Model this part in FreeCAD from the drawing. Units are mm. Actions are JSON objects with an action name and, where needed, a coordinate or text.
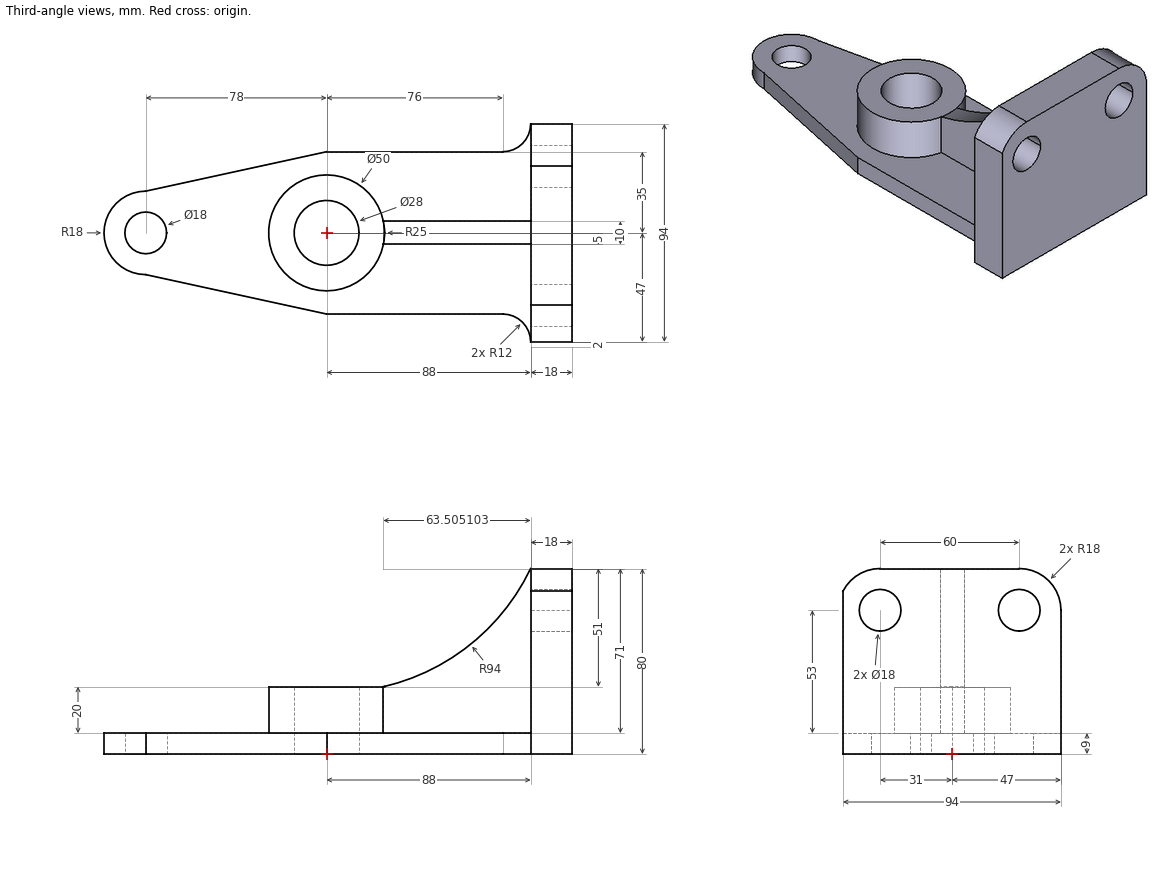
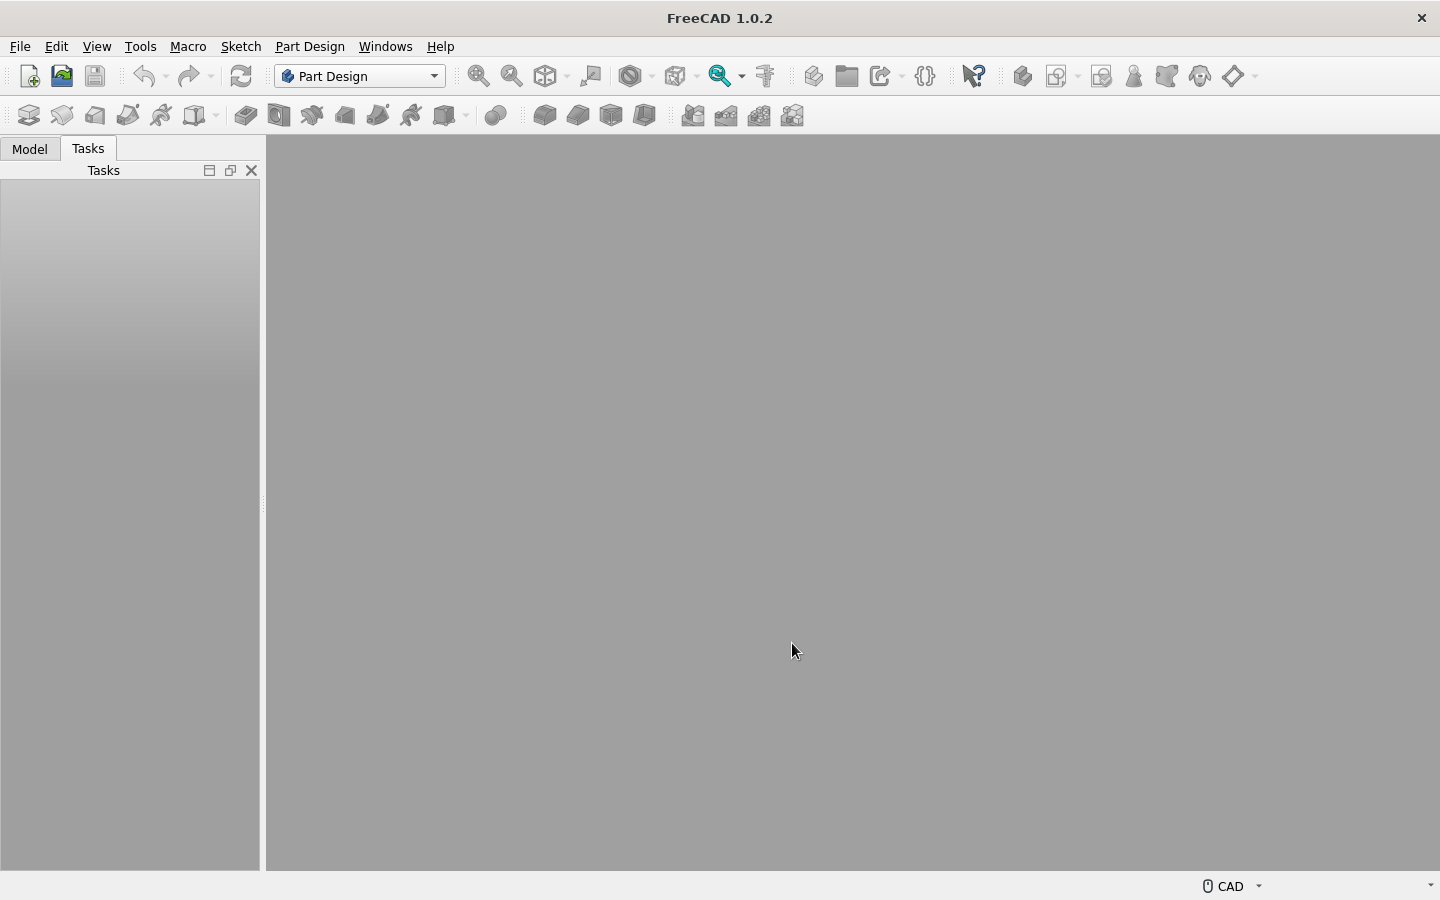
{"action": "left_click", "coordinate": [29, 76]}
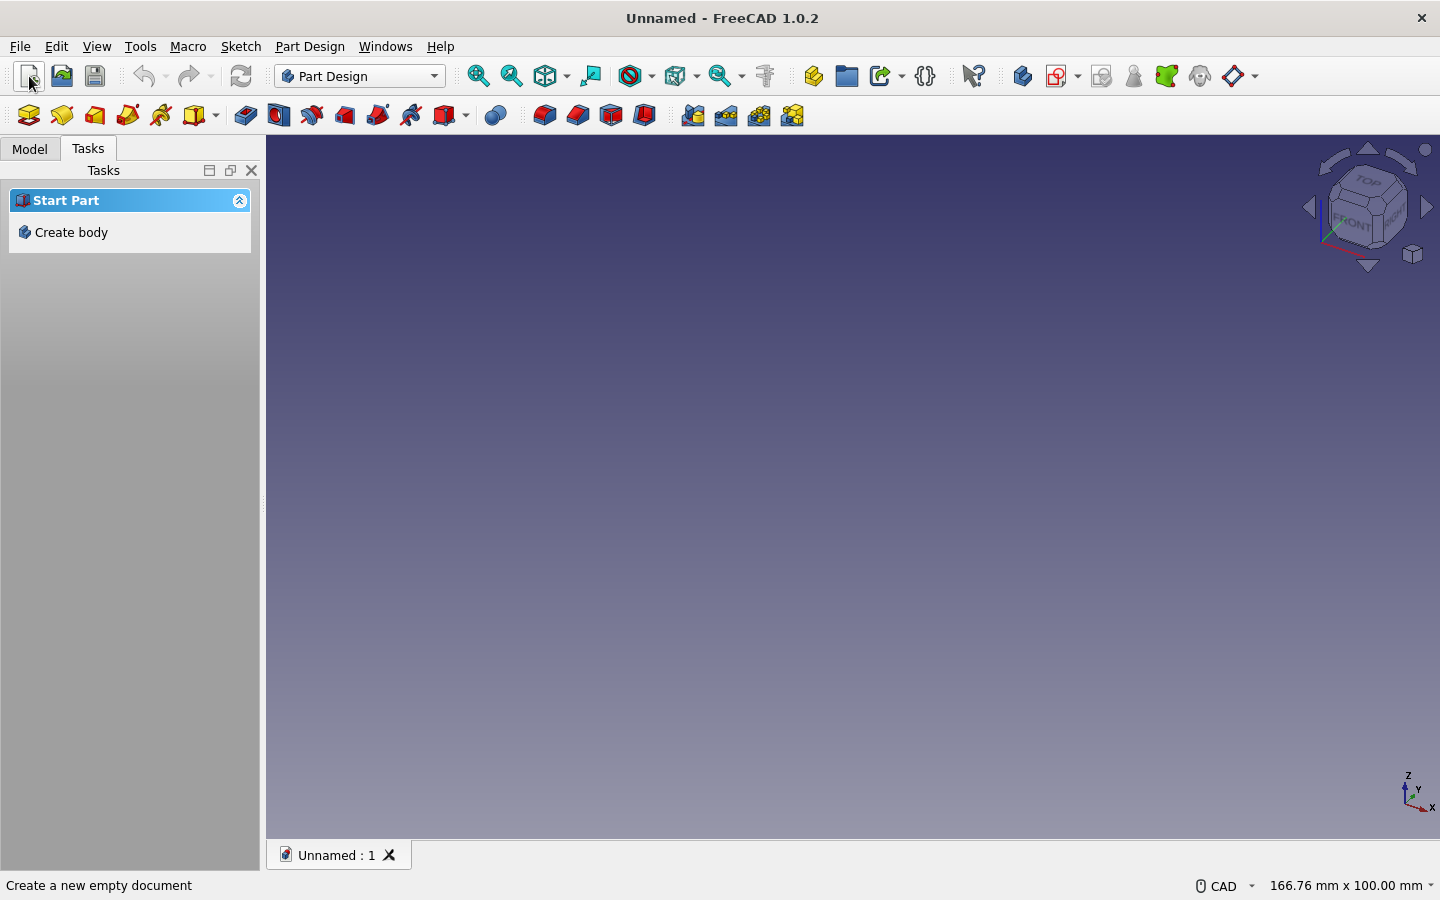
{"action": "left_click", "coordinate": [1056, 76]}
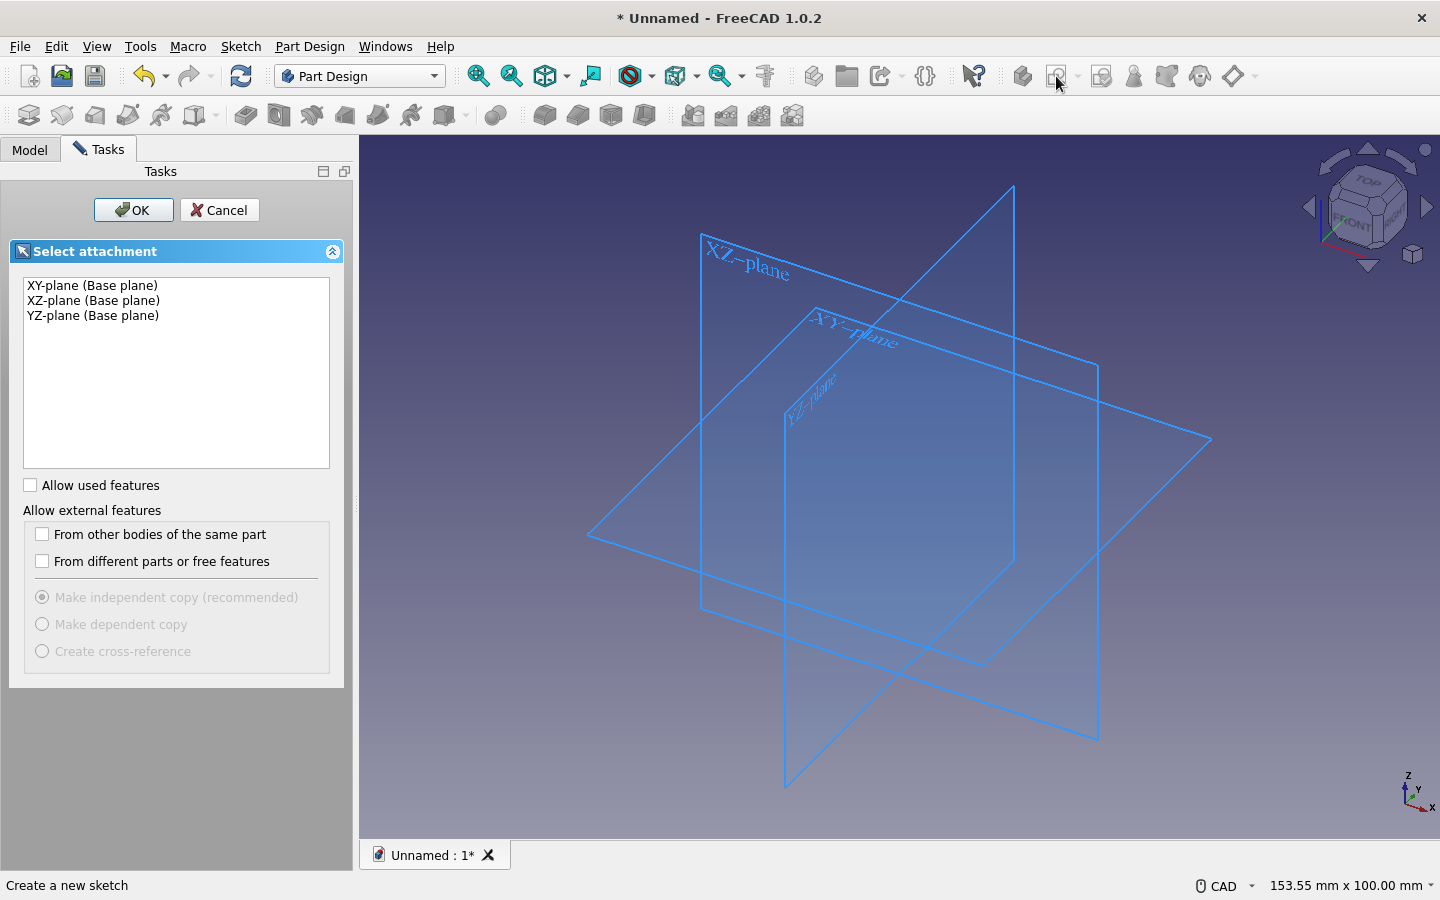
{"action": "left_click", "coordinate": [84, 286]}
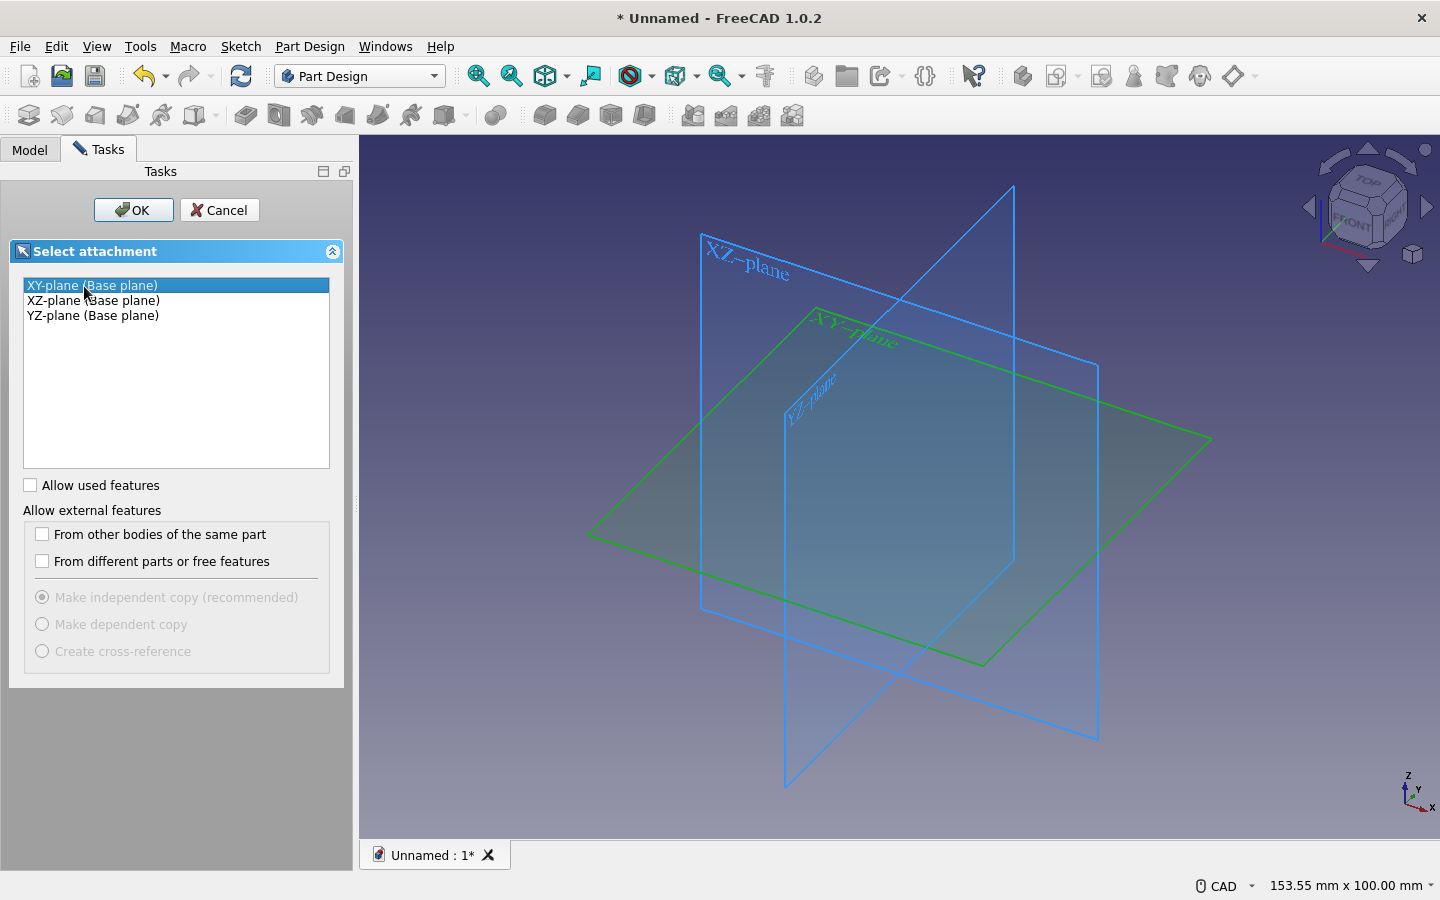
{"action": "left_click", "coordinate": [134, 210]}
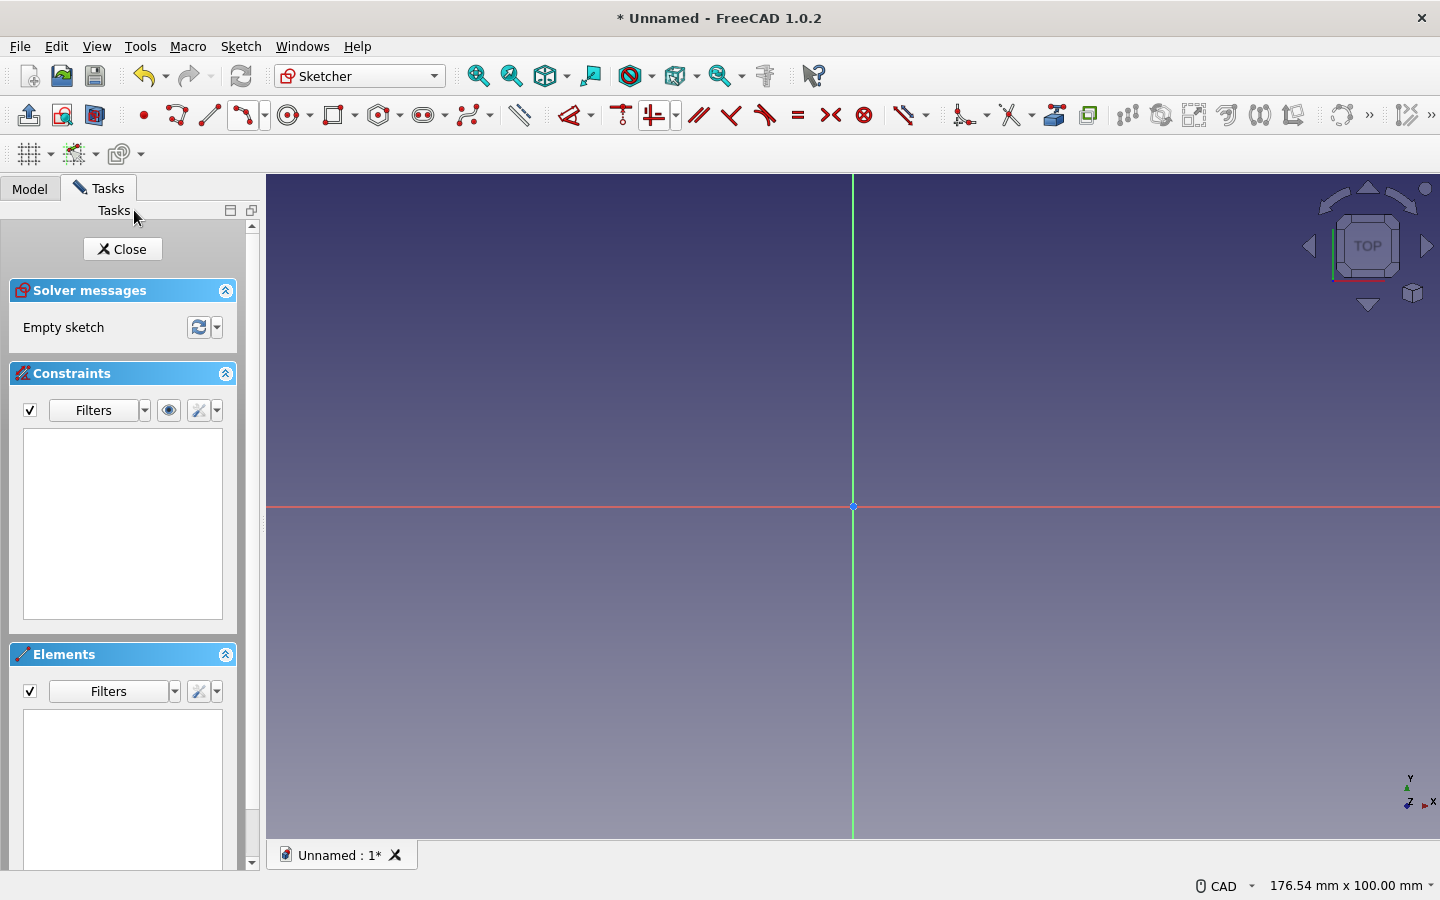
{"action": "scroll", "coordinate": [734, 506], "scroll_direction": "down", "scroll_amount": 3}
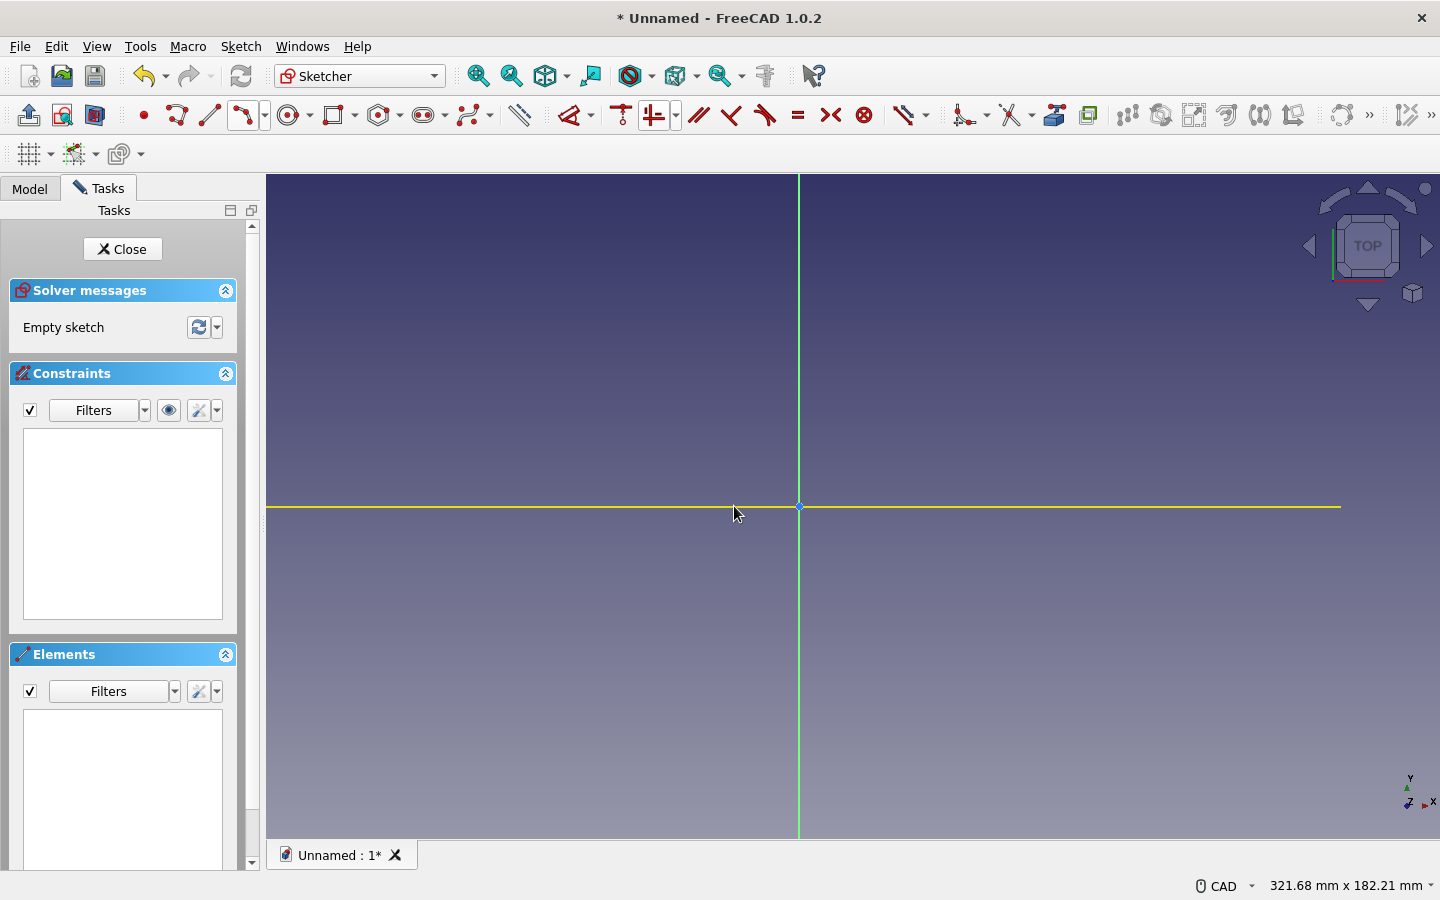
{"action": "left_click", "coordinate": [177, 116]}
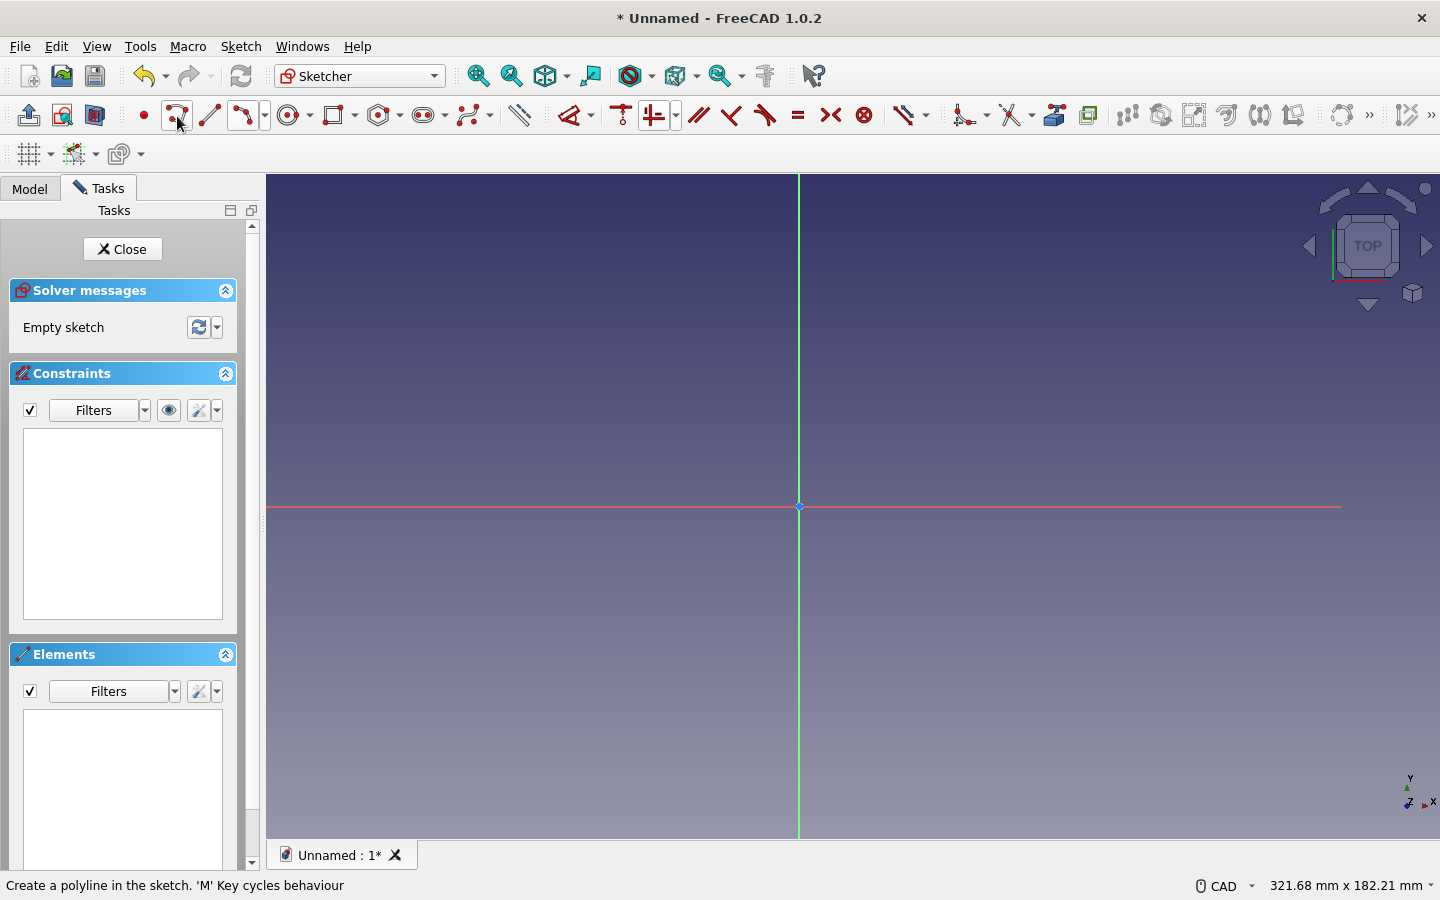
{"action": "left_click", "coordinate": [1077, 379]}
{"action": "left_click", "coordinate": [799, 379]}
{"action": "left_click", "coordinate": [515, 441]}
{"action": "right_click", "coordinate": [515, 441]}